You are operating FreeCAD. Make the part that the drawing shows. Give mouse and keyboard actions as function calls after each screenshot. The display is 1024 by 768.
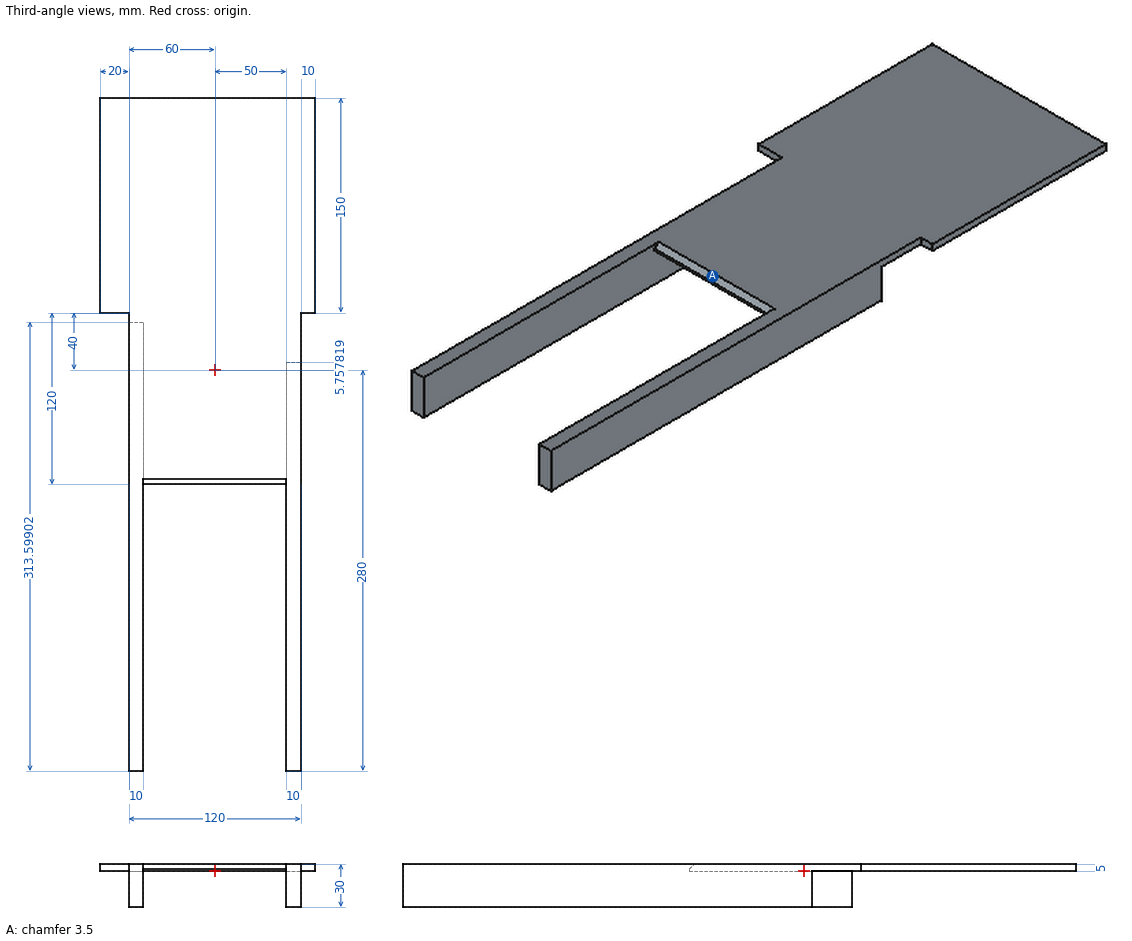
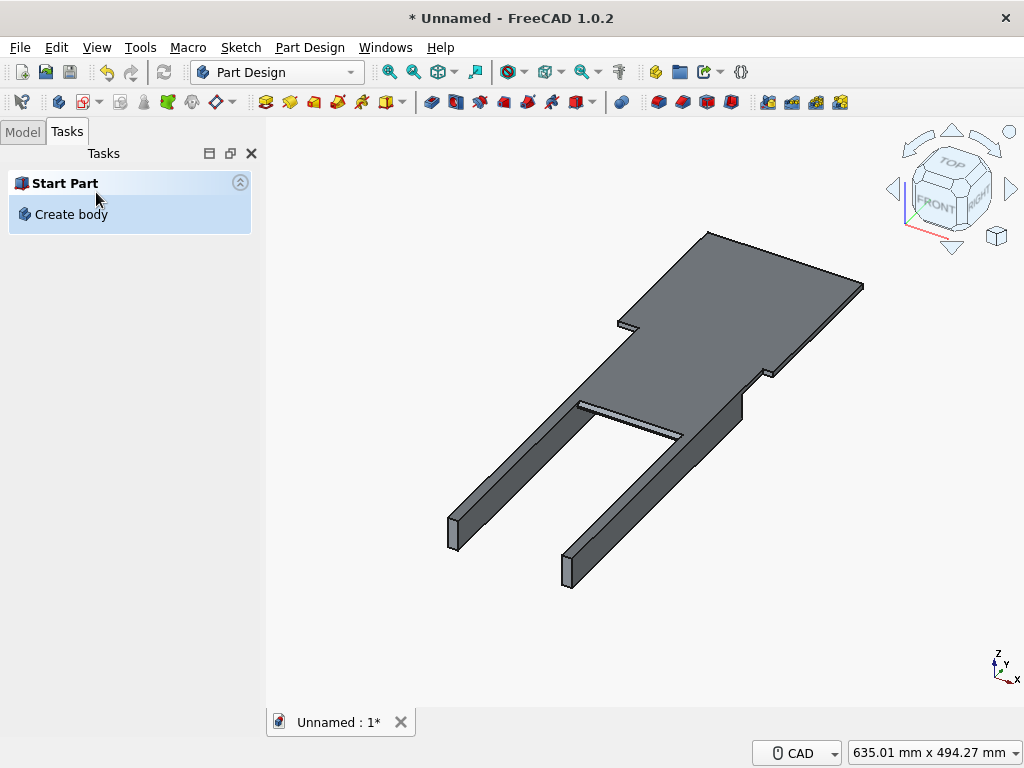
key(0)